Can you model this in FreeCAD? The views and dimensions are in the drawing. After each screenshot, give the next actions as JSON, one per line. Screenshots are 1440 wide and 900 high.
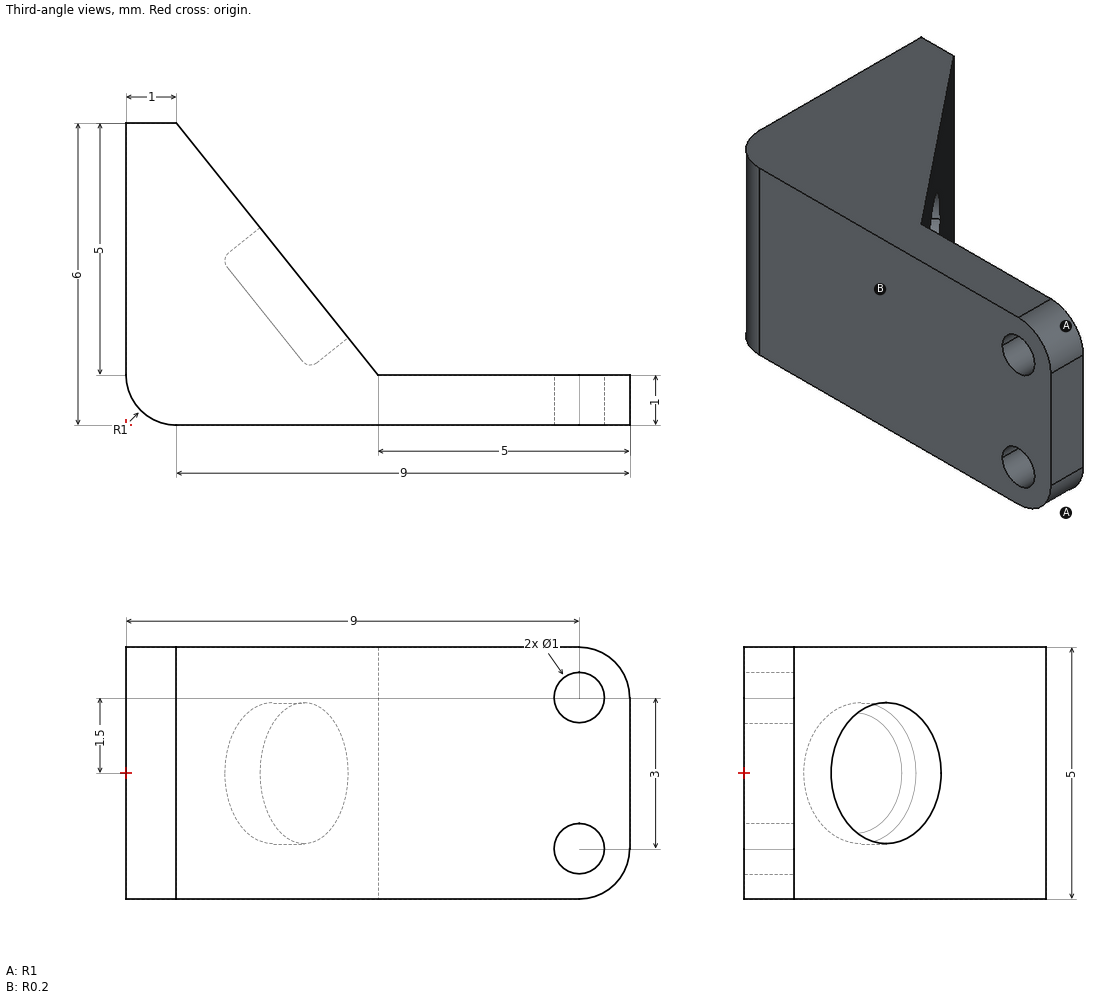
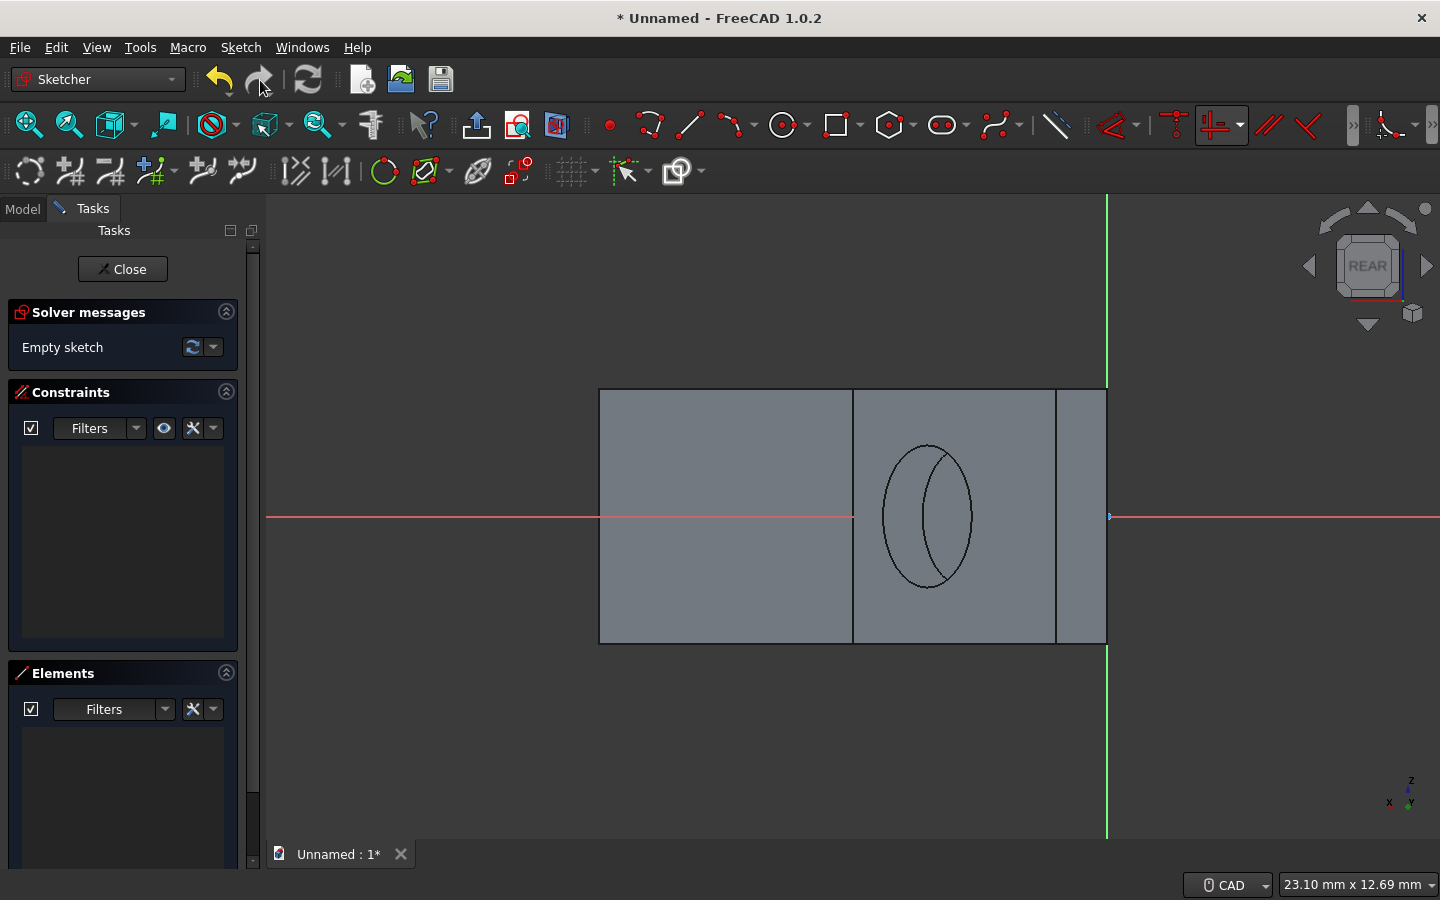
{"action": "left_click", "coordinate": [558, 126]}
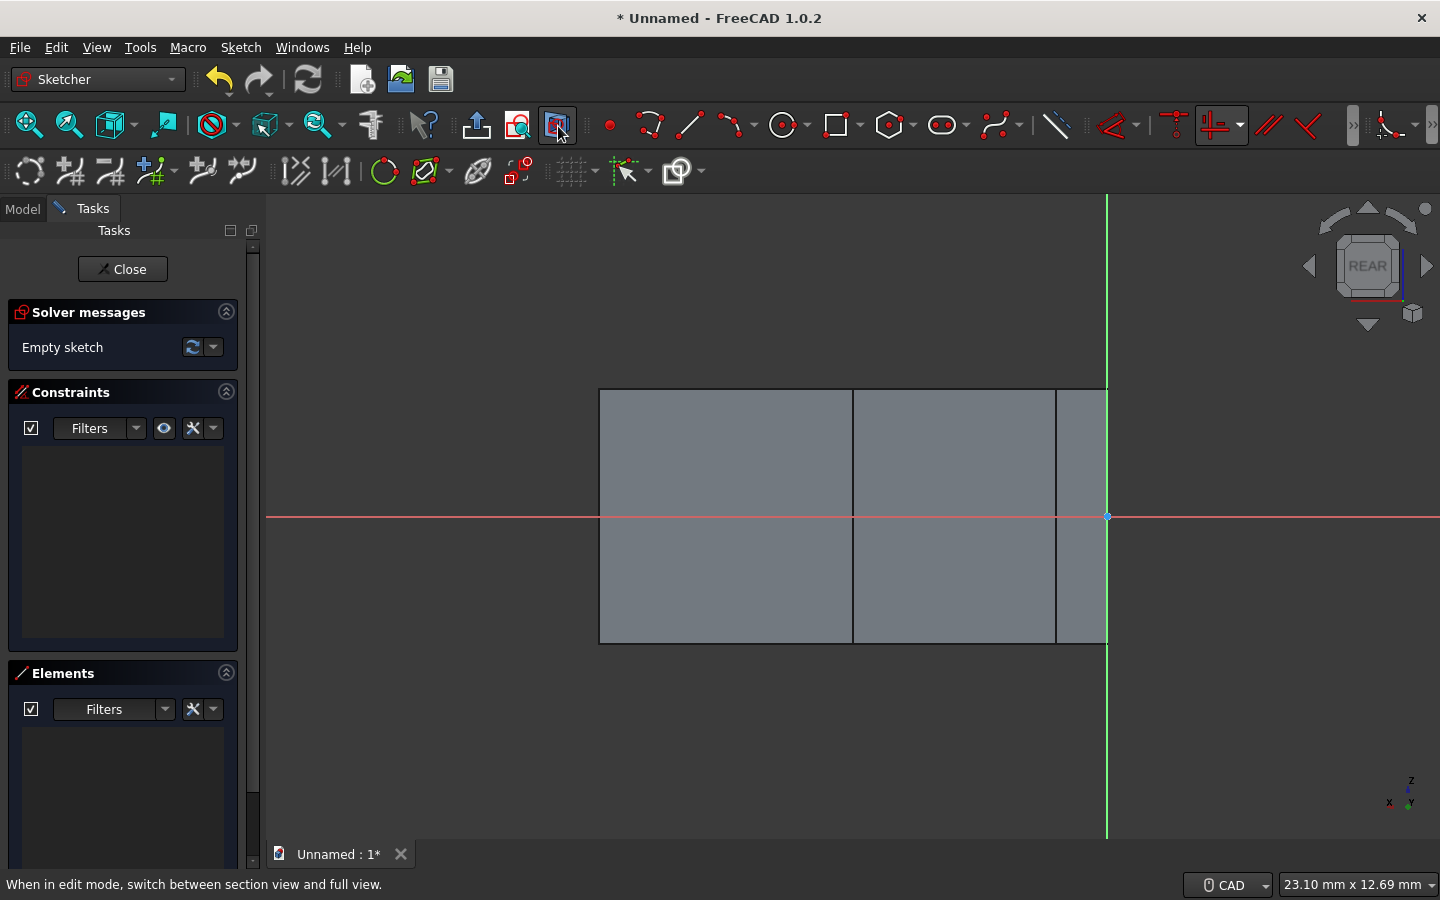
{"action": "scroll", "coordinate": [1031, 516], "scroll_direction": "up", "scroll_amount": 2}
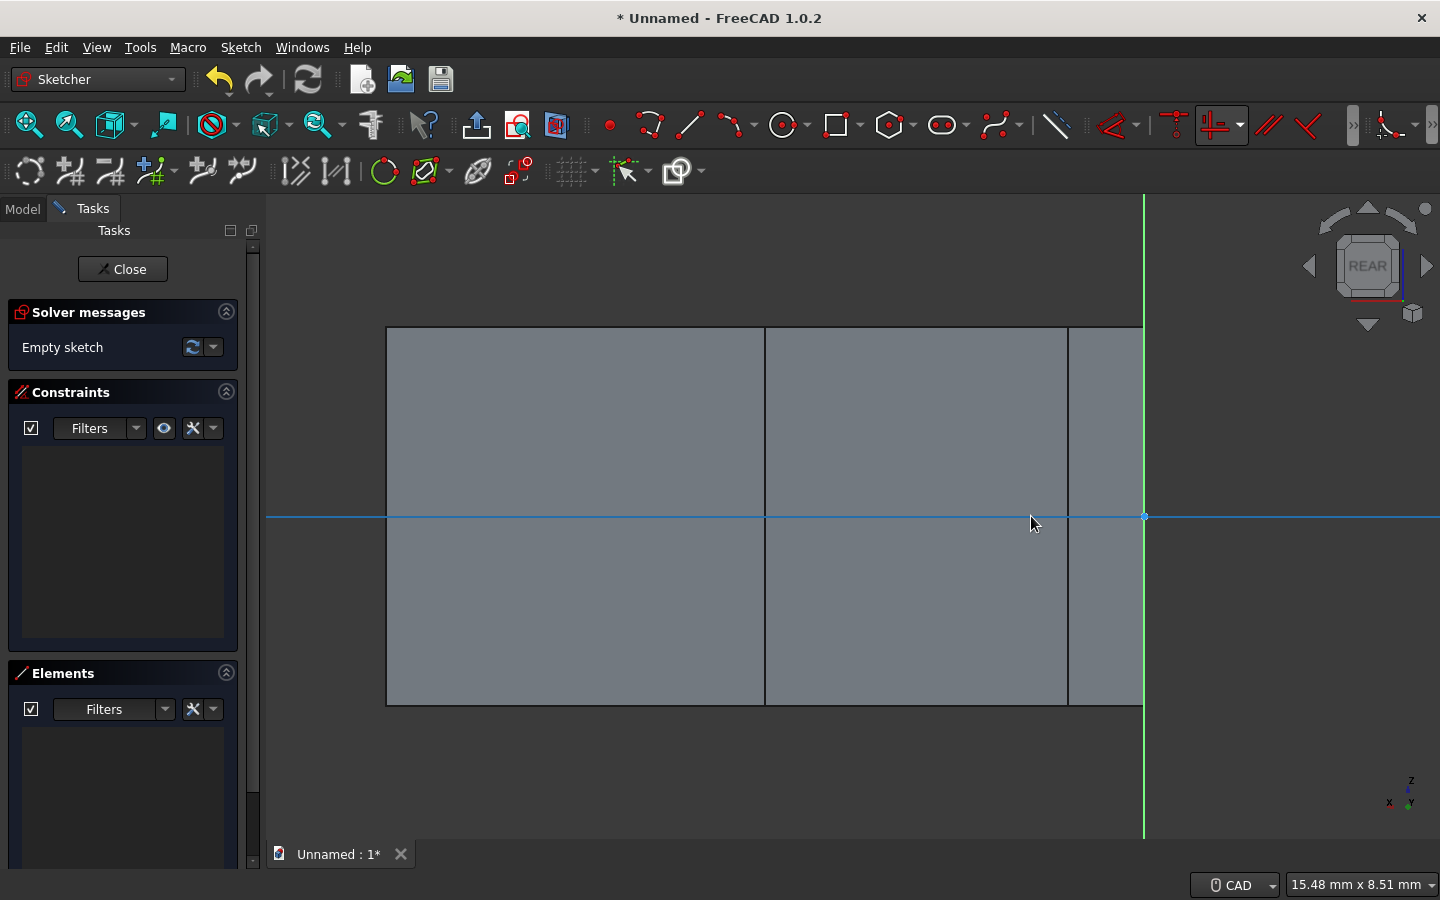
{"action": "key", "text": "g c"}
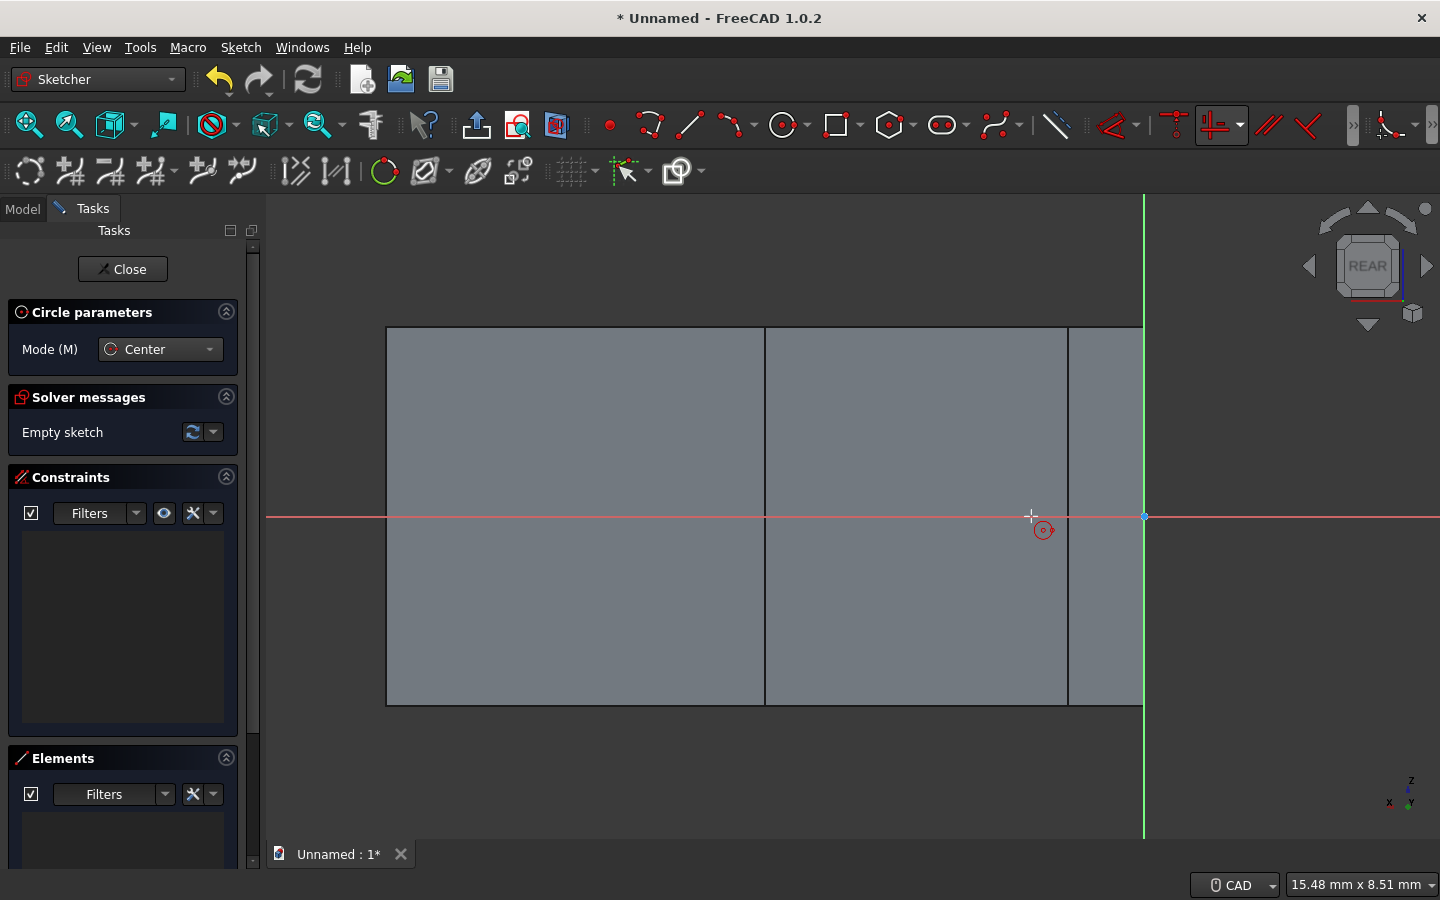
{"action": "left_click", "coordinate": [462, 403]}
{"action": "mouse_move", "coordinate": [489, 376]}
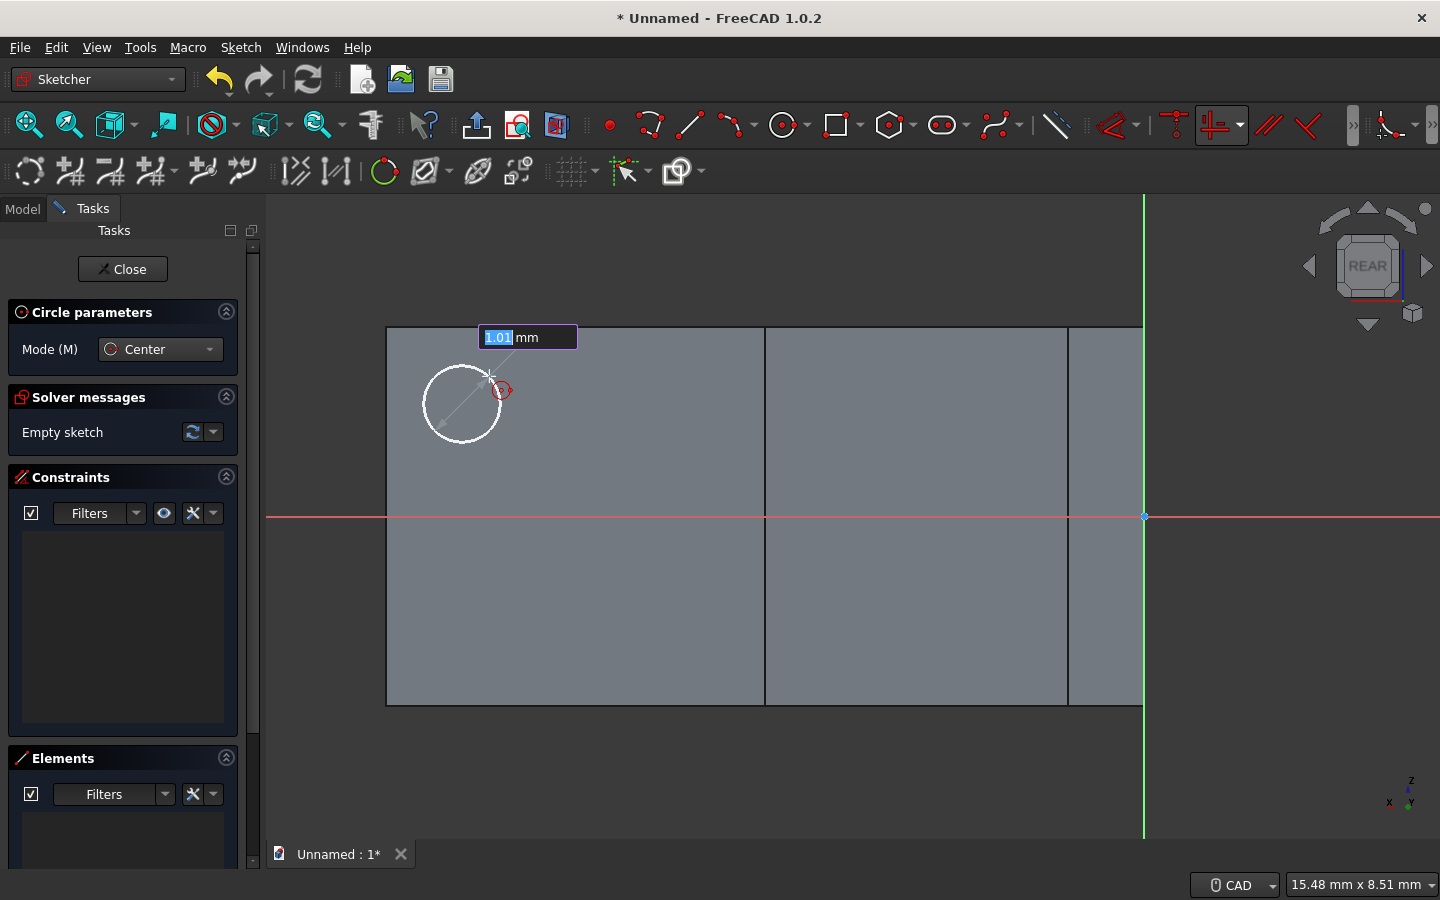
{"action": "type", "text": "1"}
{"action": "key", "text": "Return"}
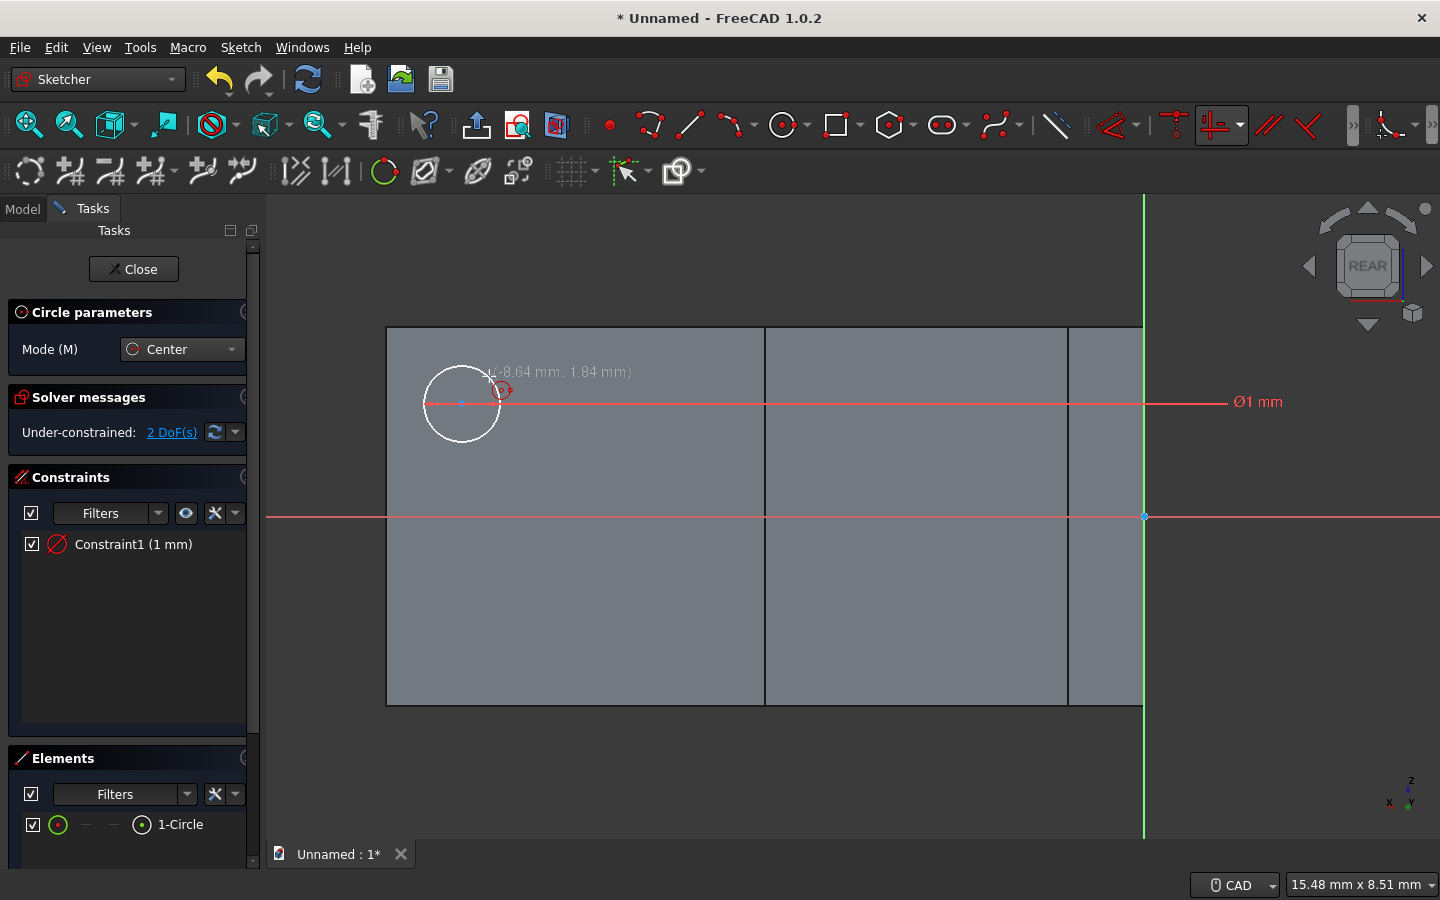
{"action": "left_click", "coordinate": [462, 630]}
{"action": "mouse_move", "coordinate": [489, 603]}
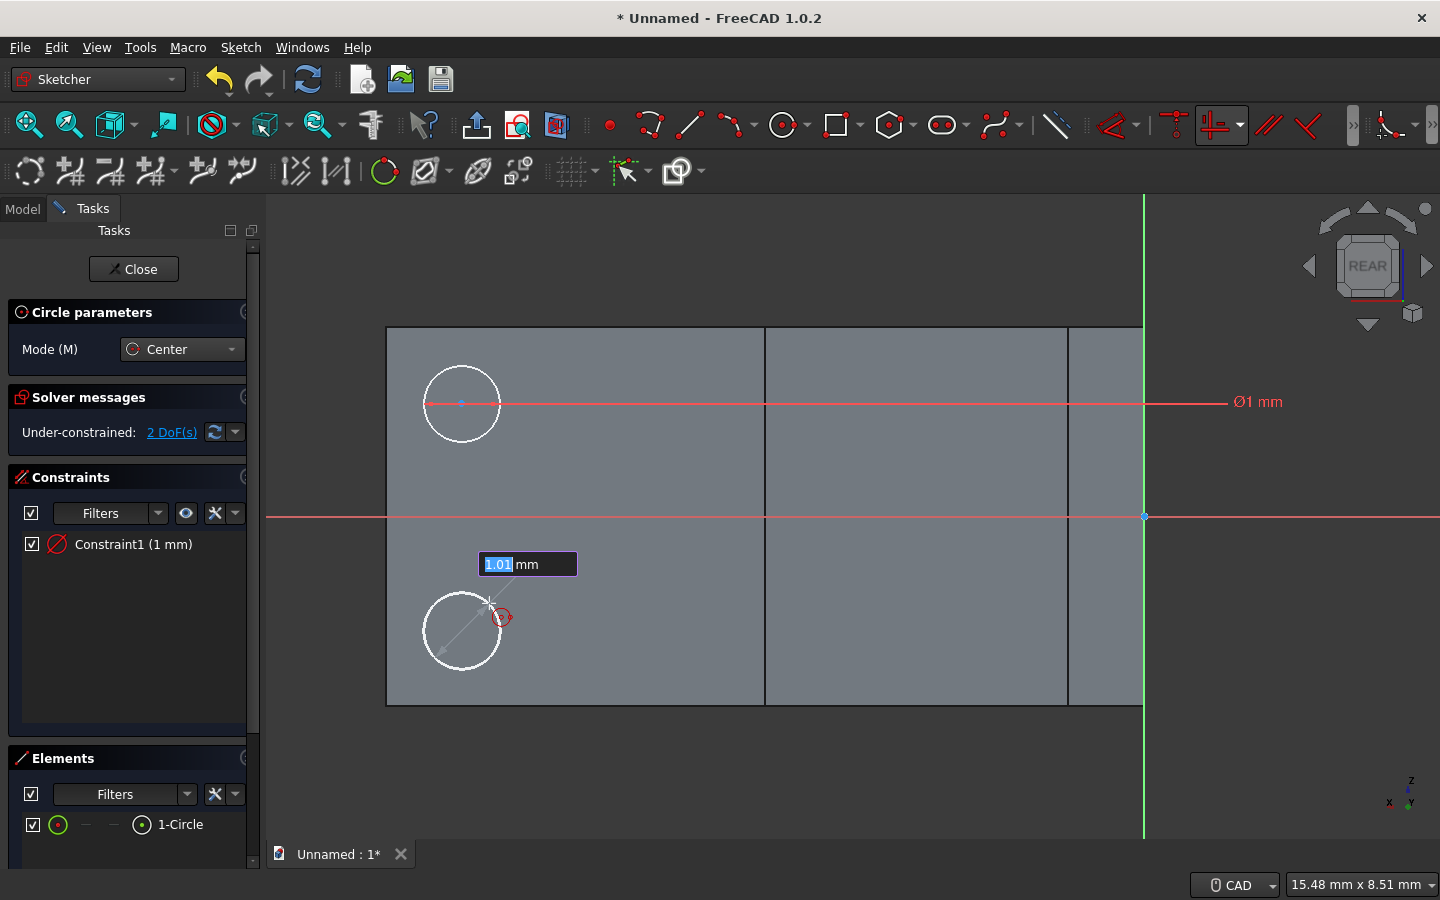
{"action": "type", "text": "1"}
{"action": "key", "text": "Return"}
{"action": "key", "text": "Escape"}